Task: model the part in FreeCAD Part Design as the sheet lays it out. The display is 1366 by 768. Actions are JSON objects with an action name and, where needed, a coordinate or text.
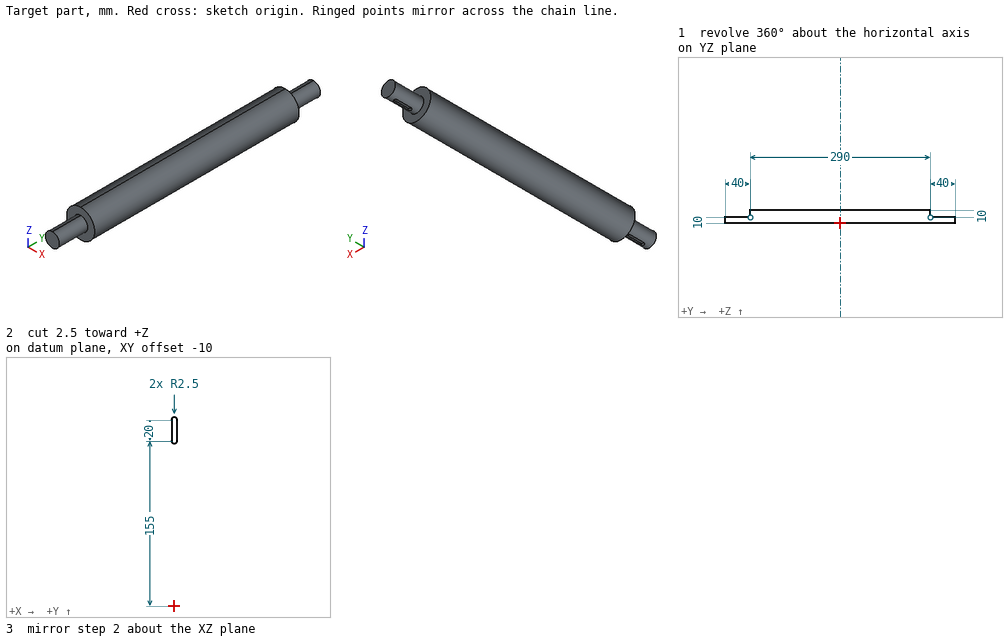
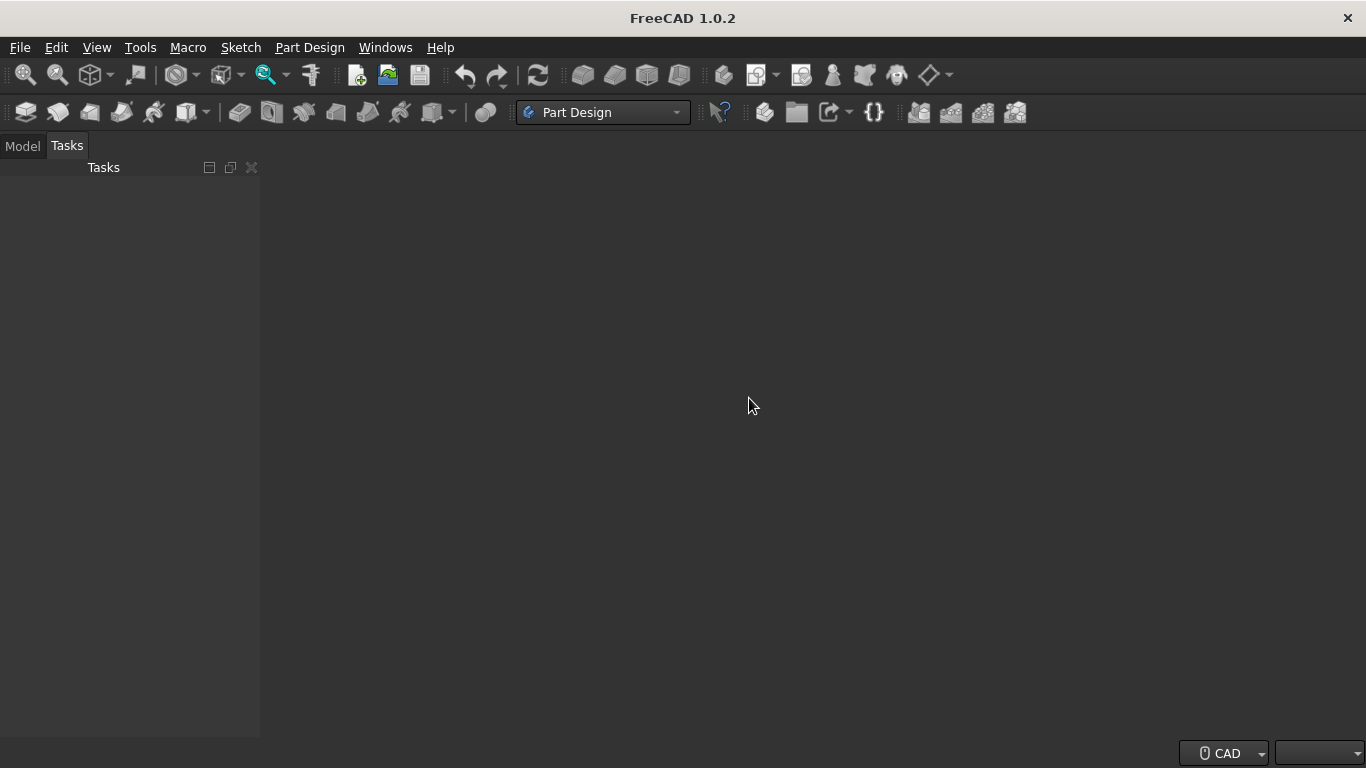
{"action": "left_click", "coordinate": [356, 76]}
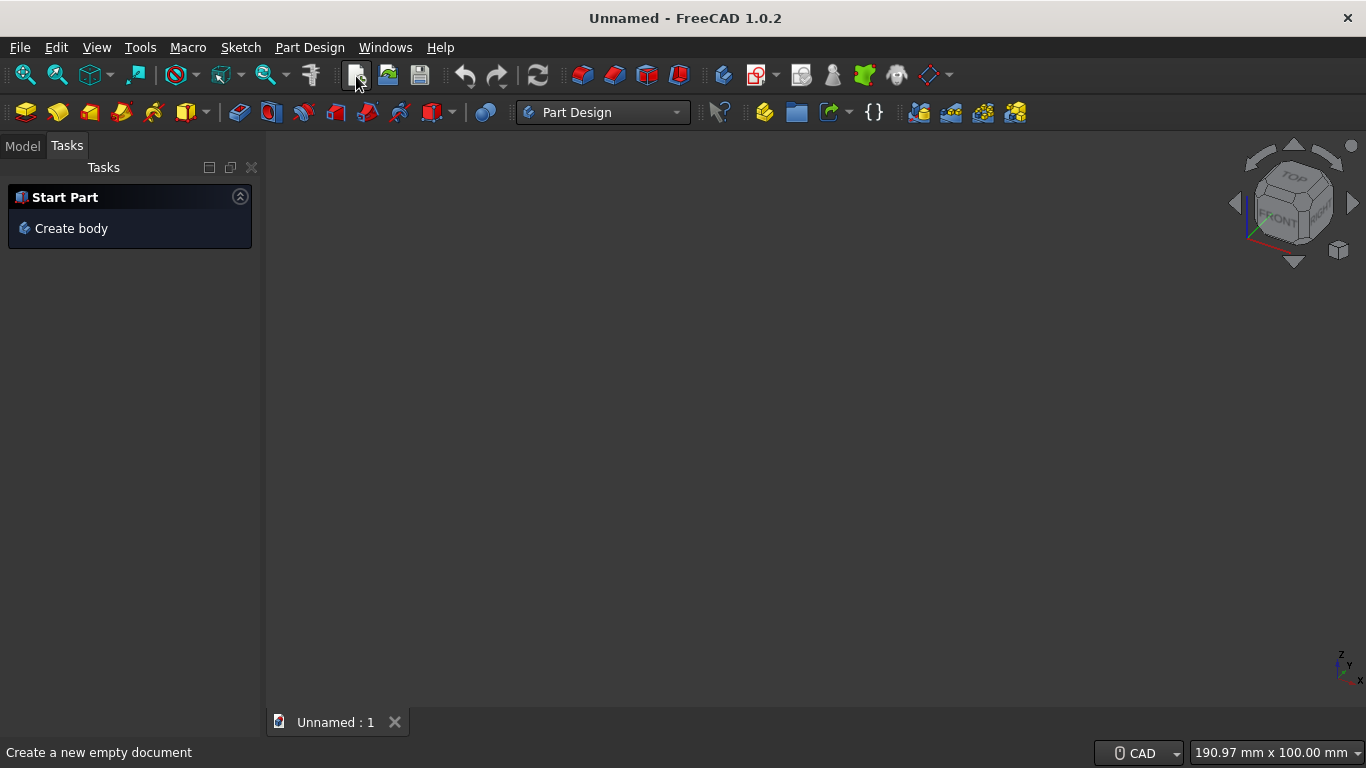
{"action": "left_click", "coordinate": [756, 76]}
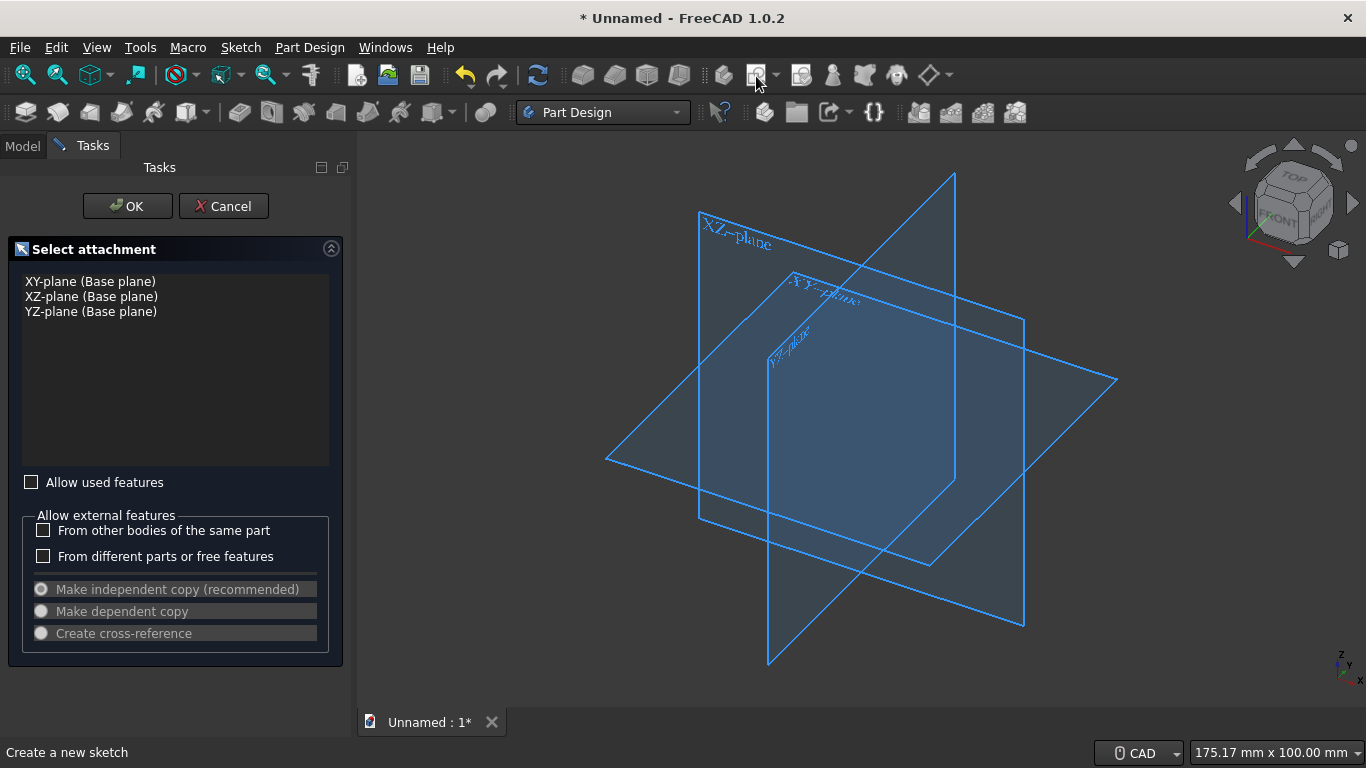
{"action": "left_click", "coordinate": [82, 312]}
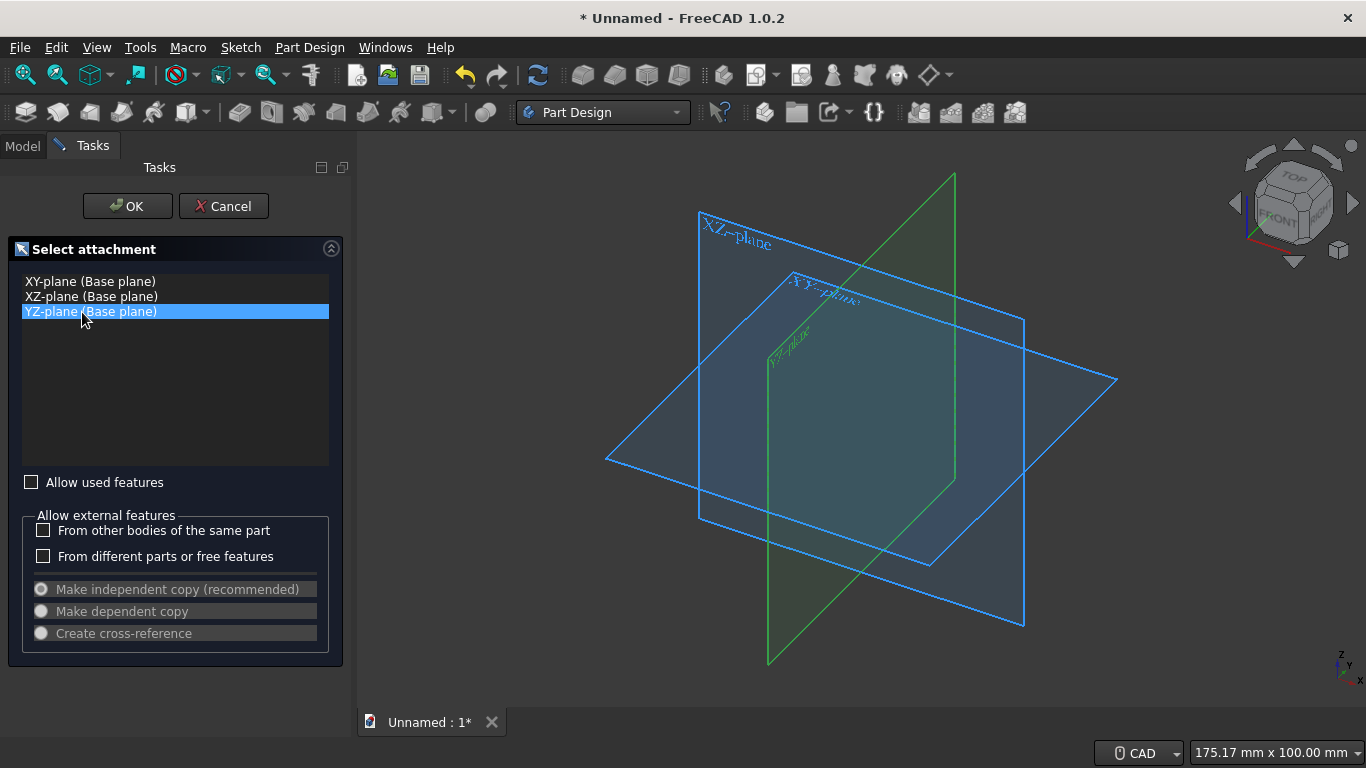
{"action": "left_click", "coordinate": [128, 206]}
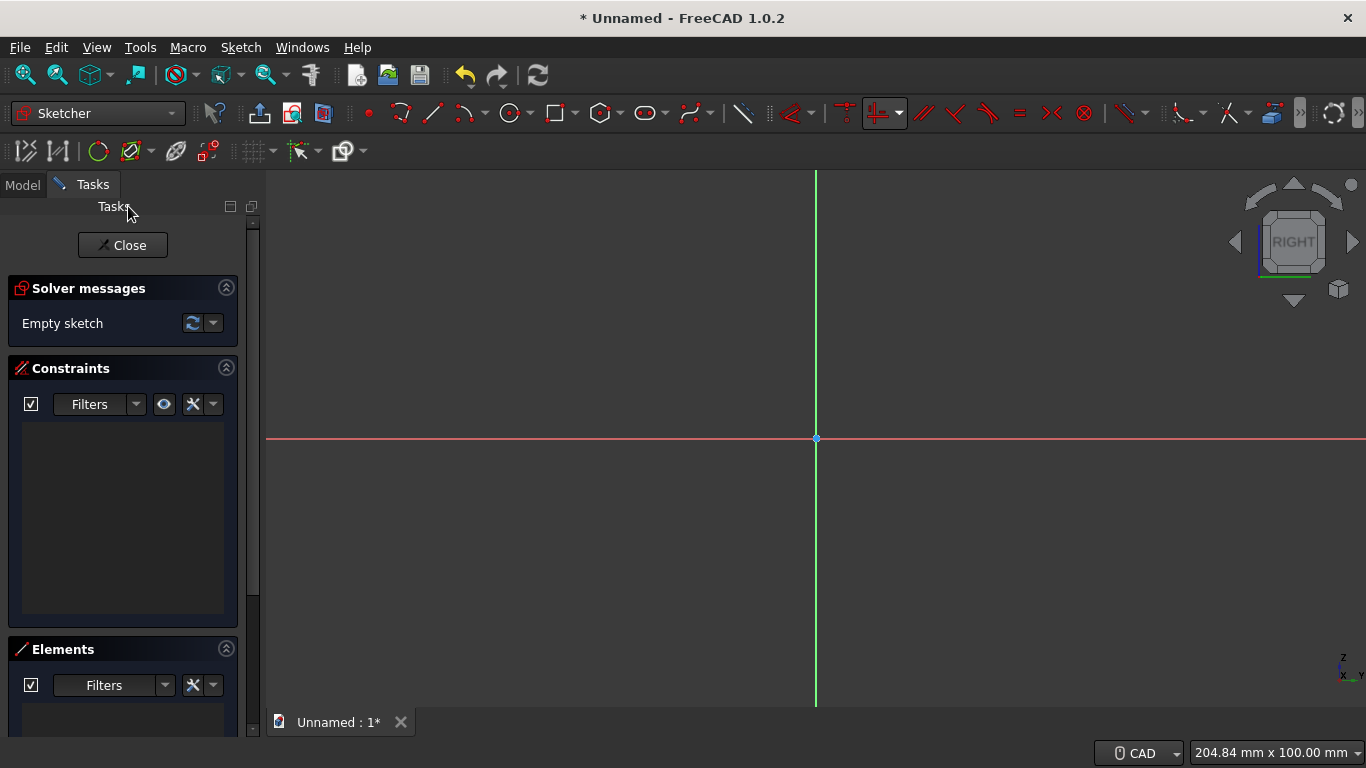
{"action": "scroll", "coordinate": [718, 462], "scroll_direction": "down", "scroll_amount": 6}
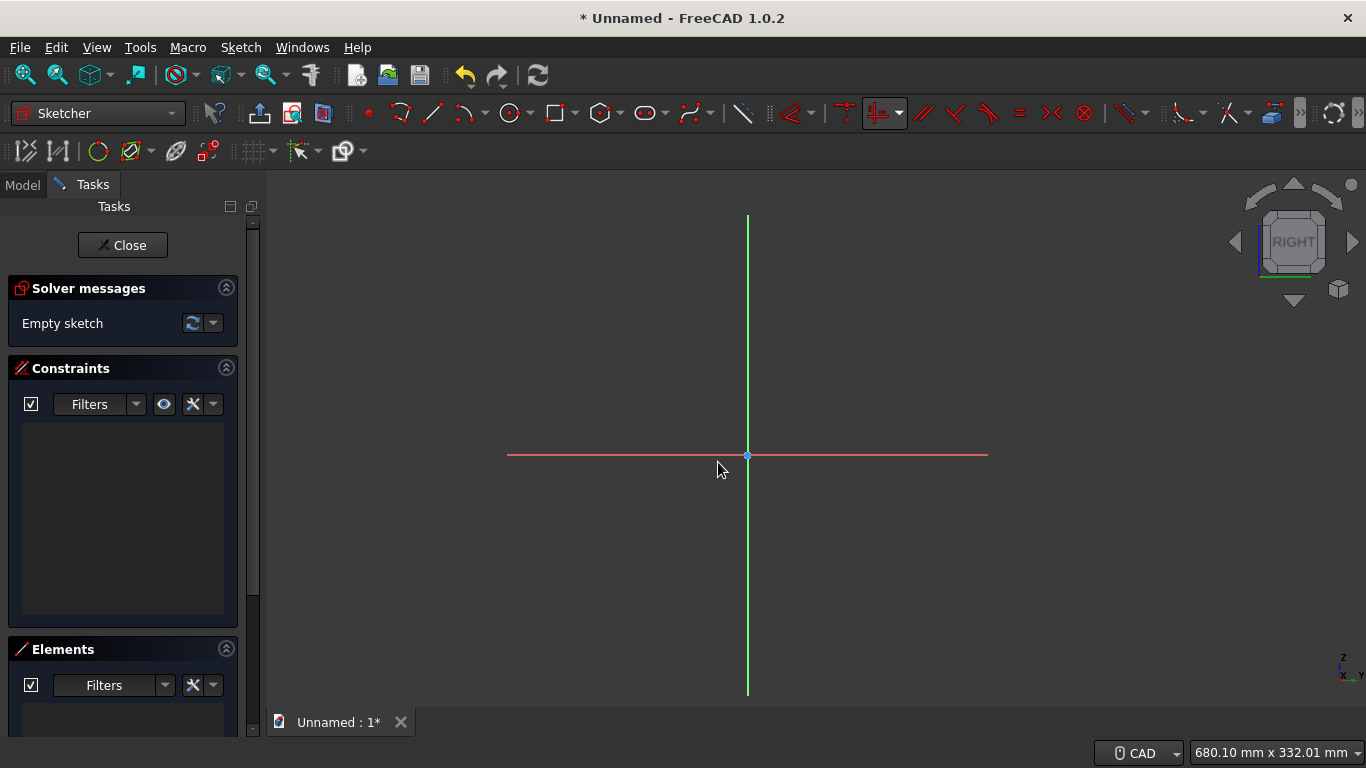
{"action": "key", "text": "g m"}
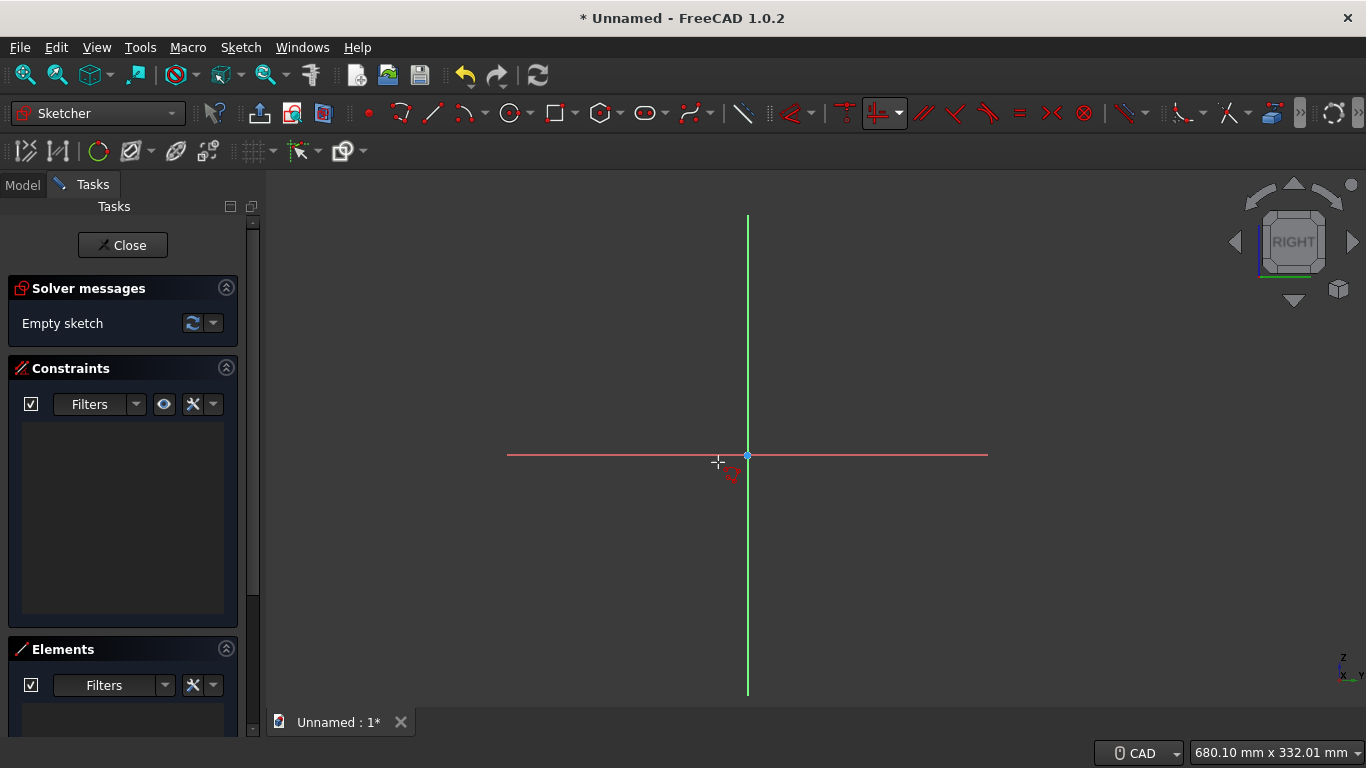
{"action": "left_click", "coordinate": [982, 439]}
{"action": "left_click", "coordinate": [982, 423]}
{"action": "left_click", "coordinate": [513, 423]}
{"action": "left_click", "coordinate": [513, 439]}
{"action": "left_click", "coordinate": [449, 439]}
{"action": "left_click", "coordinate": [449, 455]}
{"action": "left_click", "coordinate": [1047, 446]}
{"action": "left_click", "coordinate": [1047, 439]}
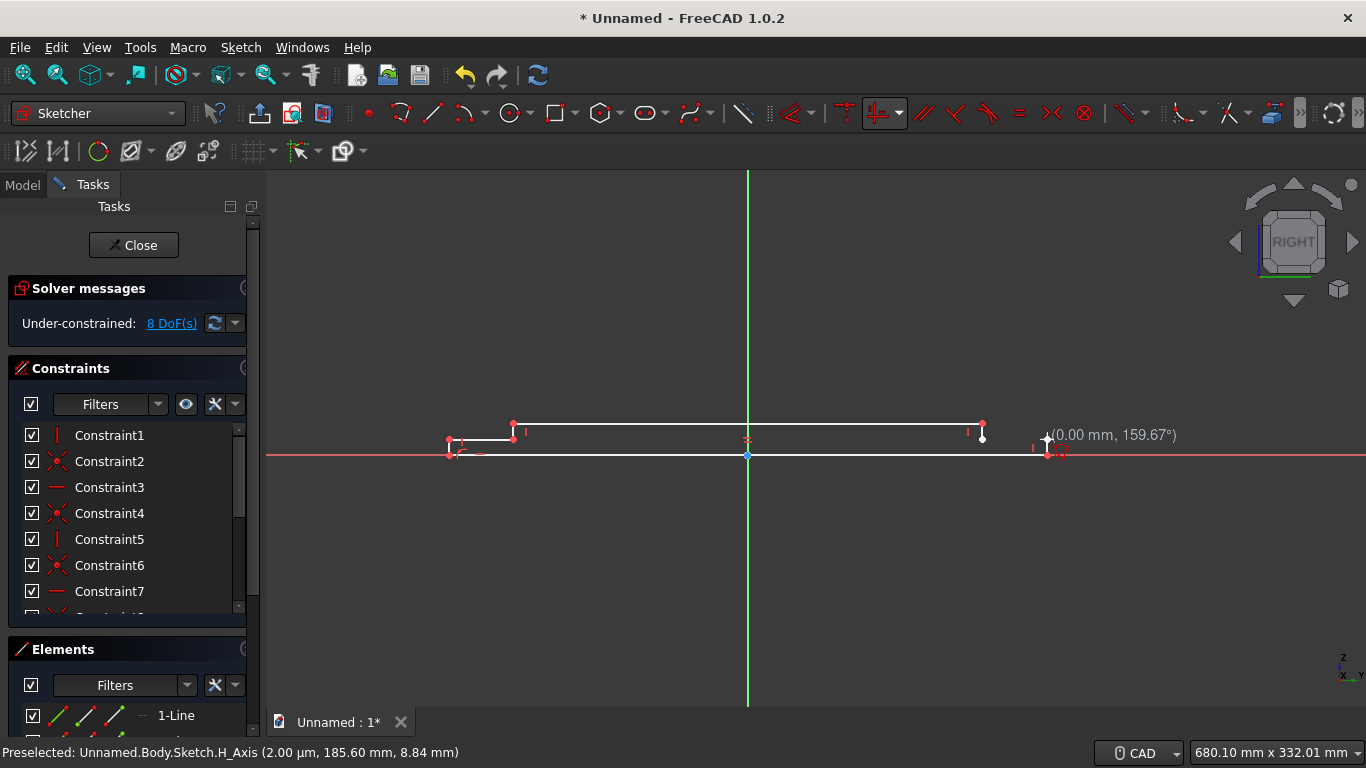
{"action": "scroll", "coordinate": [982, 439], "scroll_direction": "up", "scroll_amount": 4}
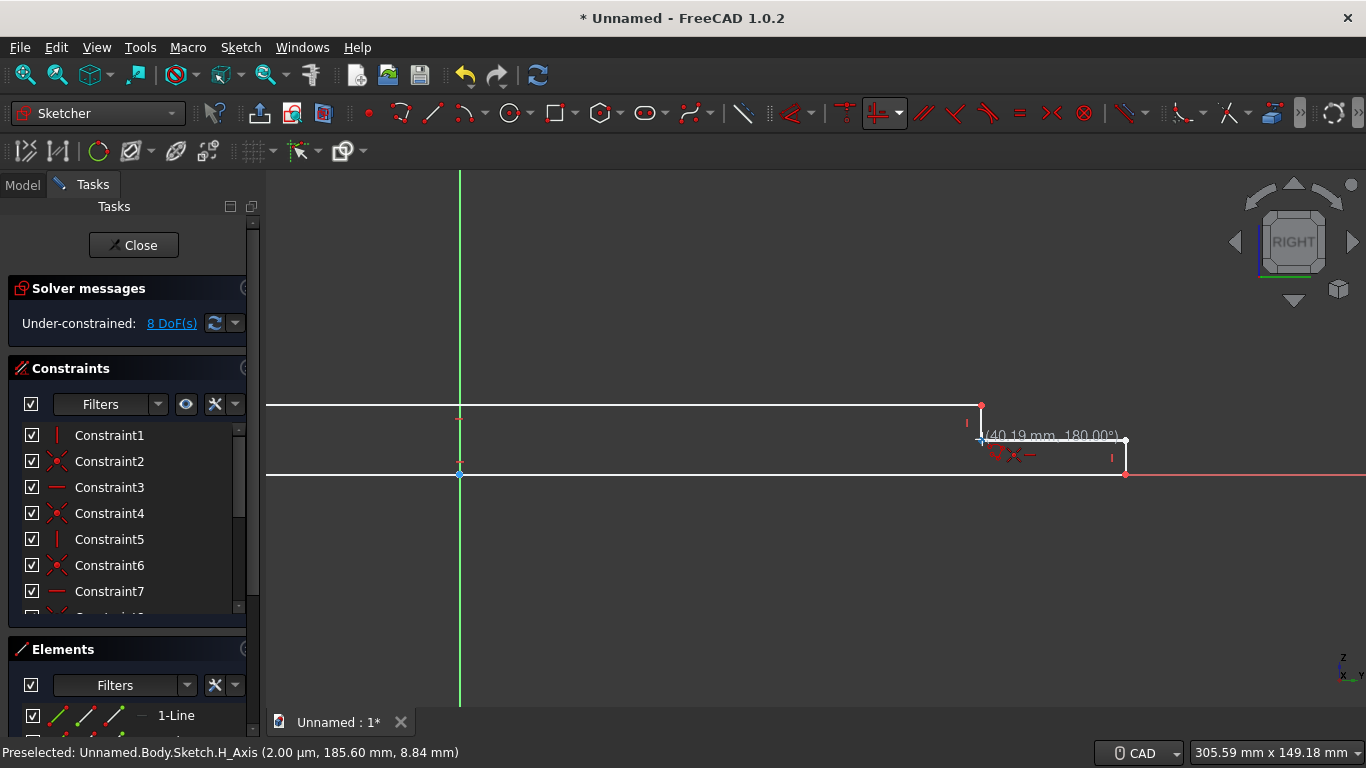
{"action": "left_click", "coordinate": [981, 441]}
{"action": "key", "text": "Escape"}
{"action": "key", "text": "Escape"}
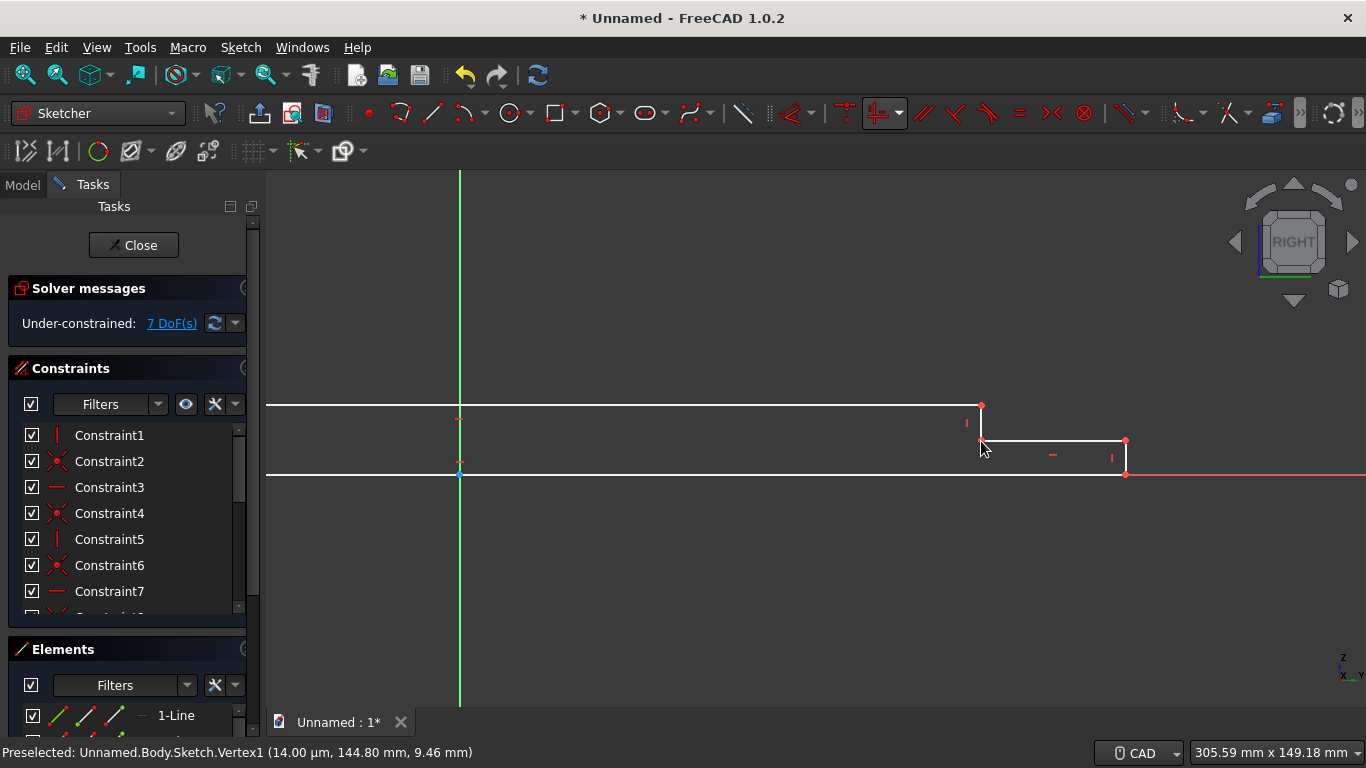
{"action": "left_click", "coordinate": [981, 441]}